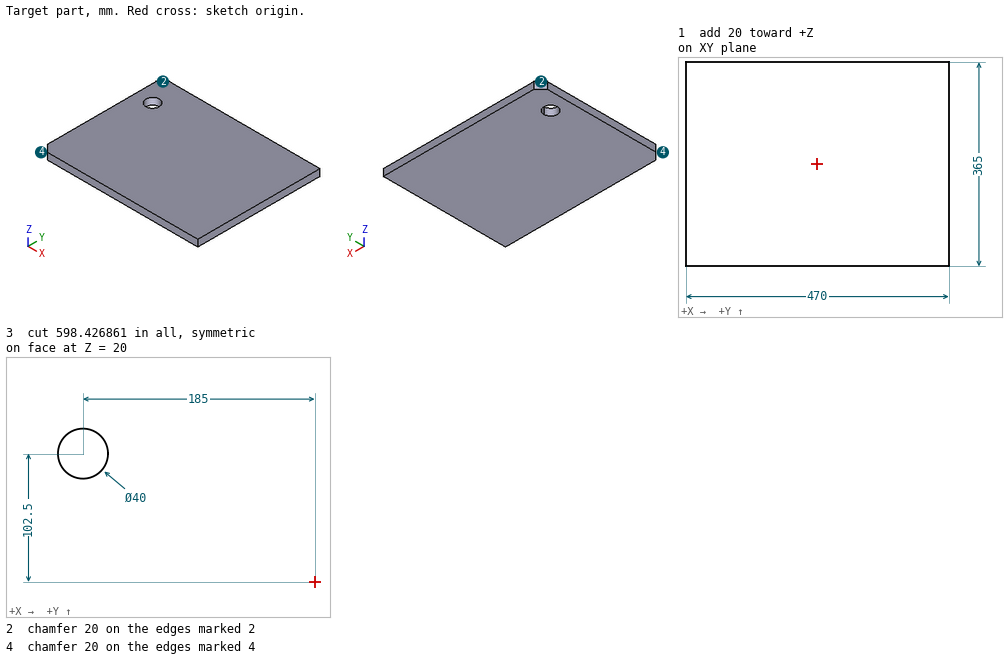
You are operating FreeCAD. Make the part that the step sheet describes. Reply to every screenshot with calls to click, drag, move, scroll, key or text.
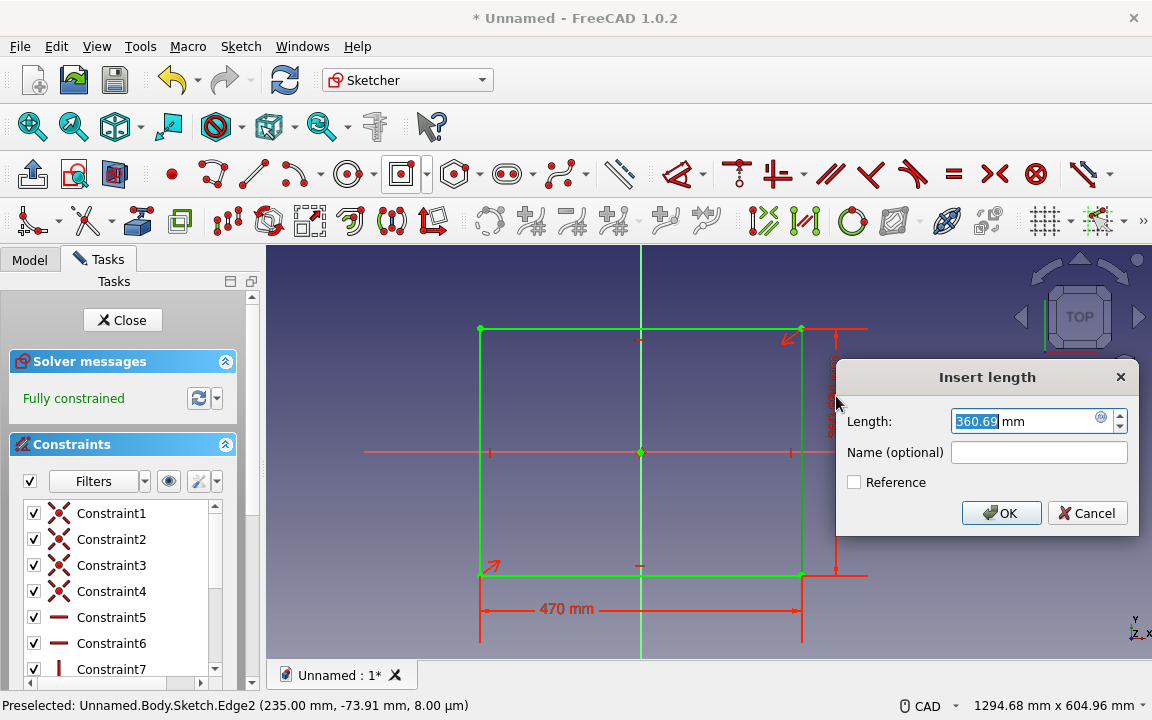
text(365)
key(Return)
key(Escape)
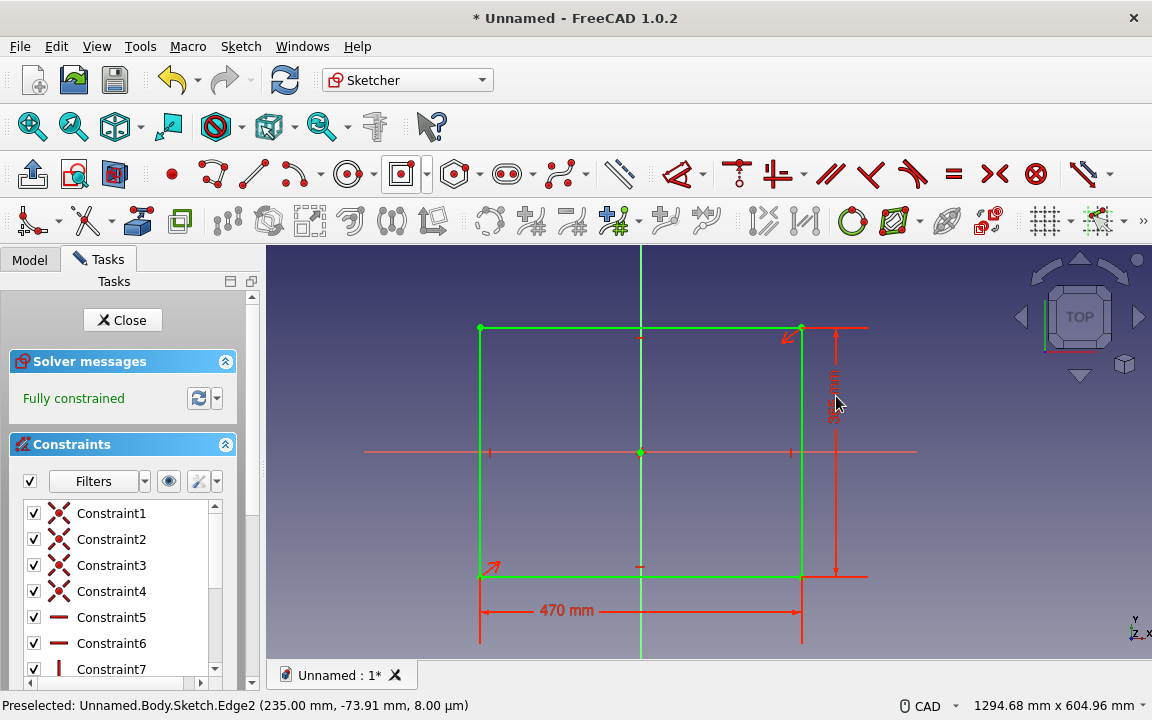
click(123, 320)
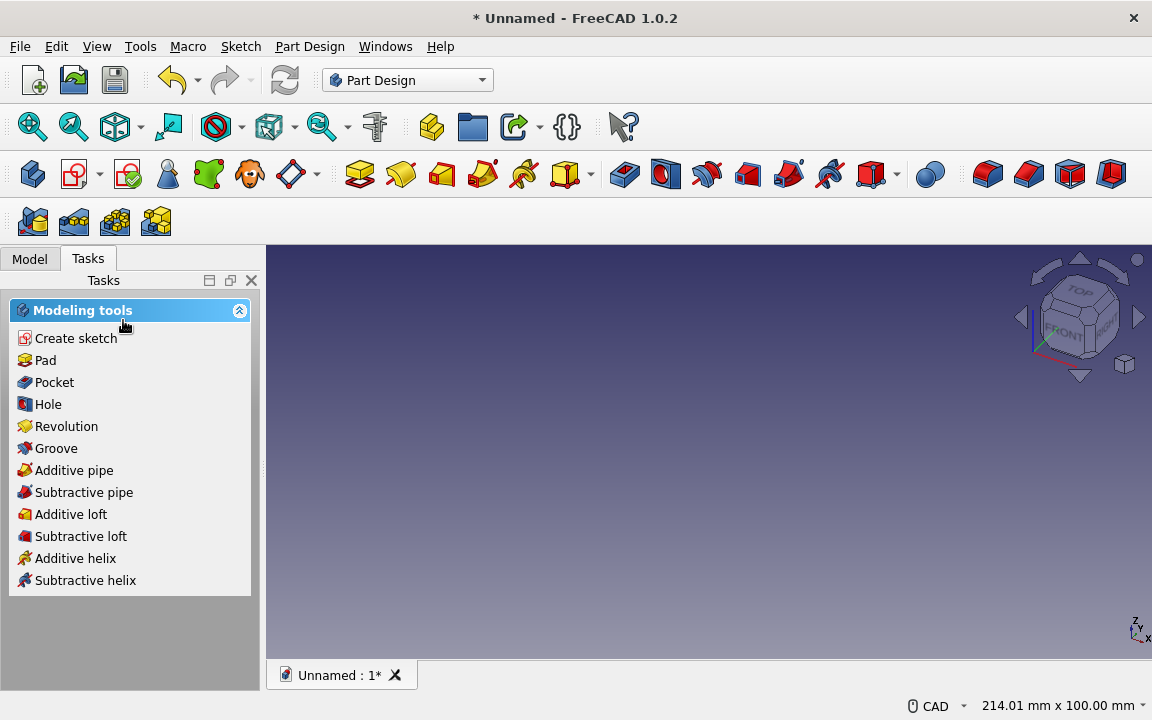
click(360, 174)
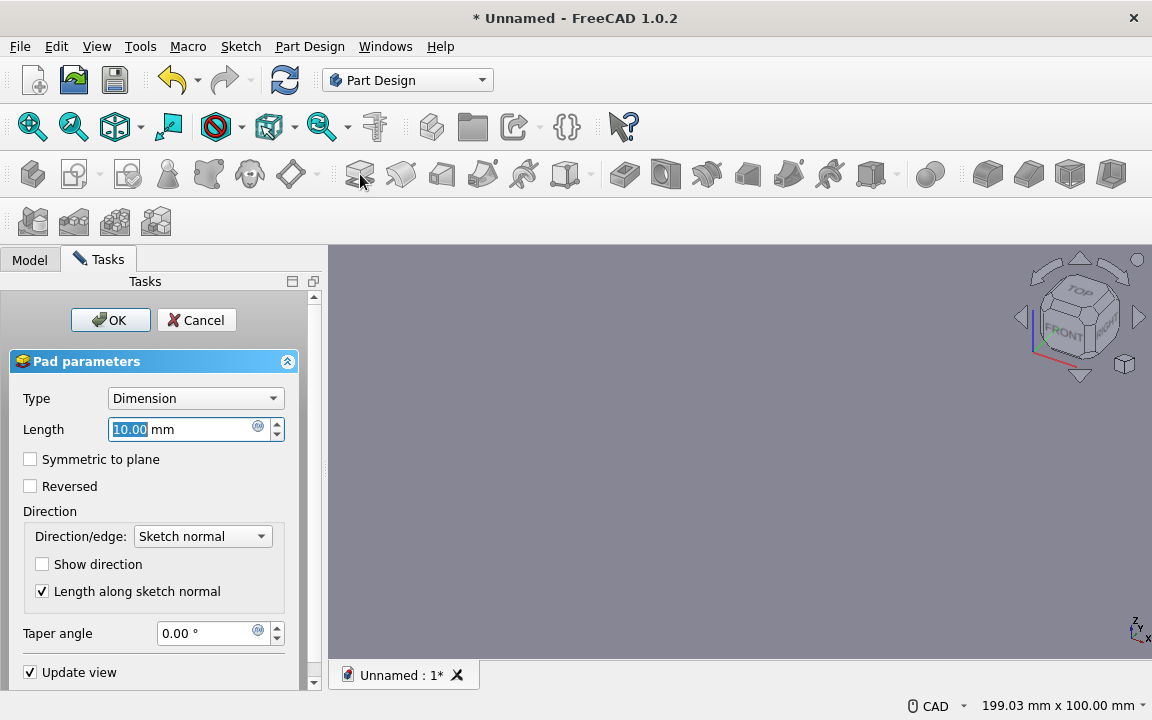
text(20)
key(Tab)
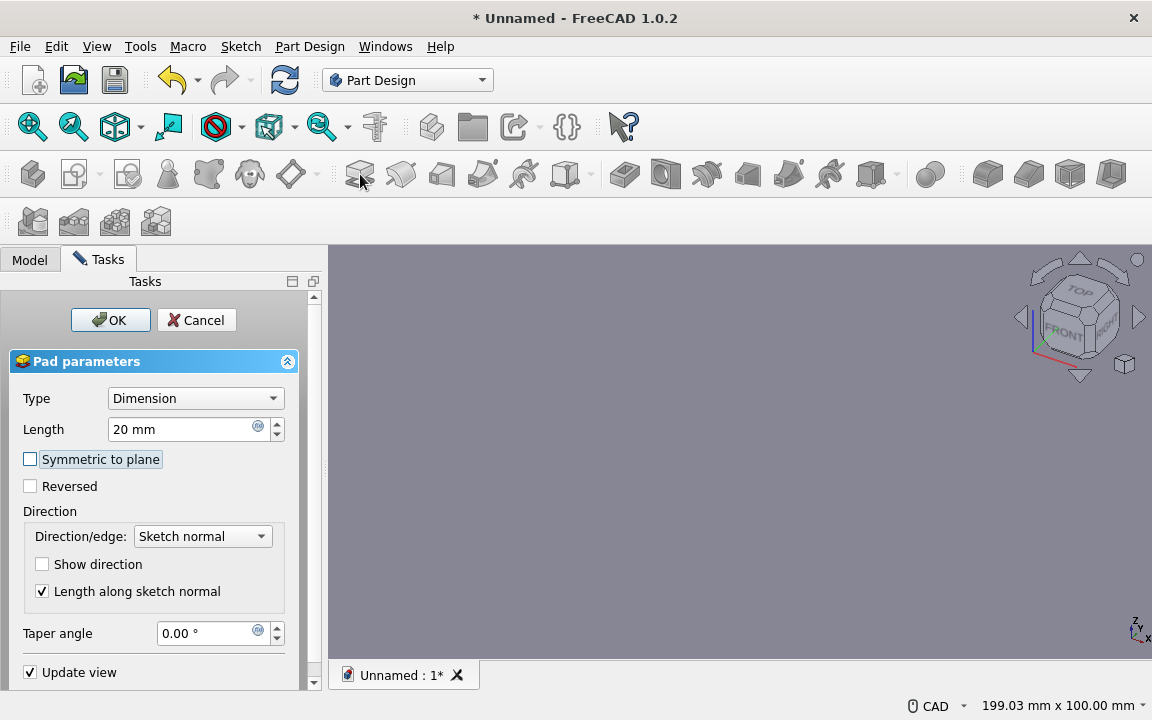
click(111, 320)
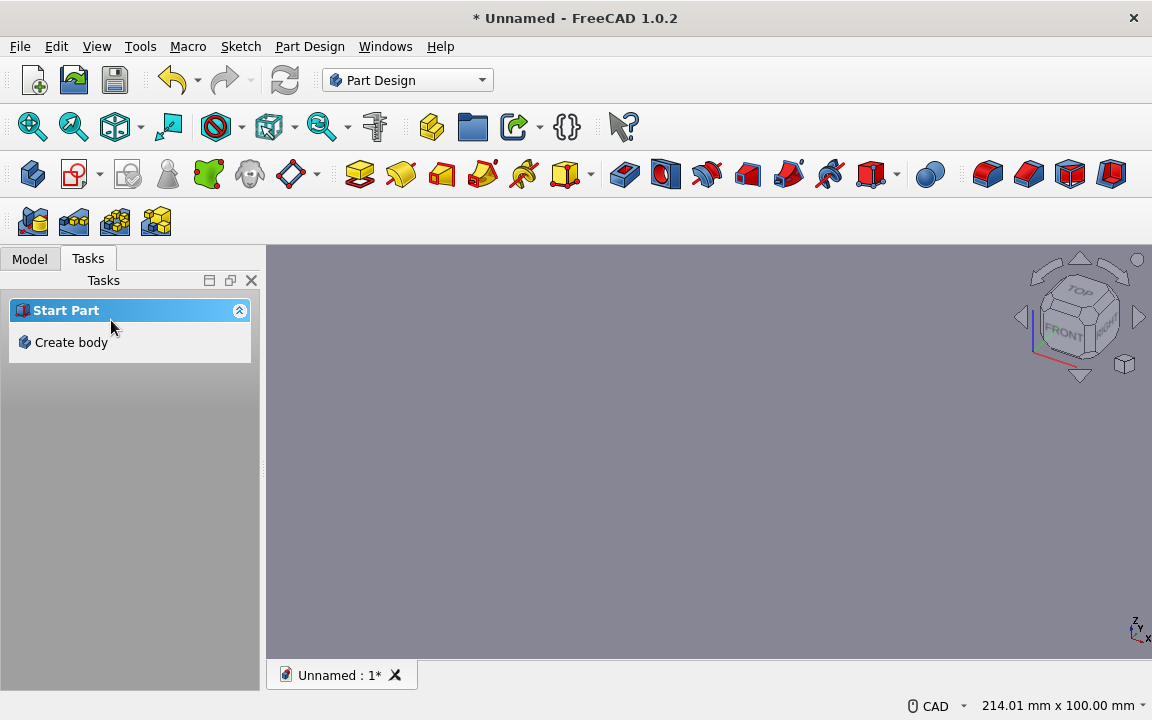
click(33, 128)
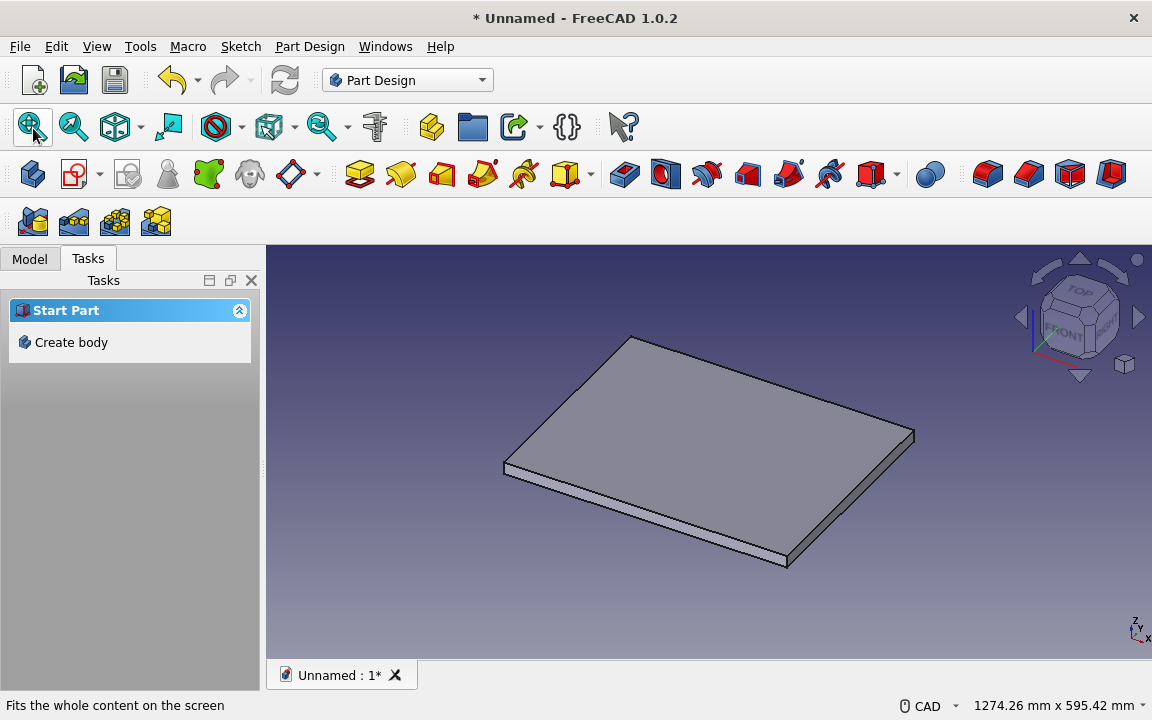
scroll(631, 341, up, 6)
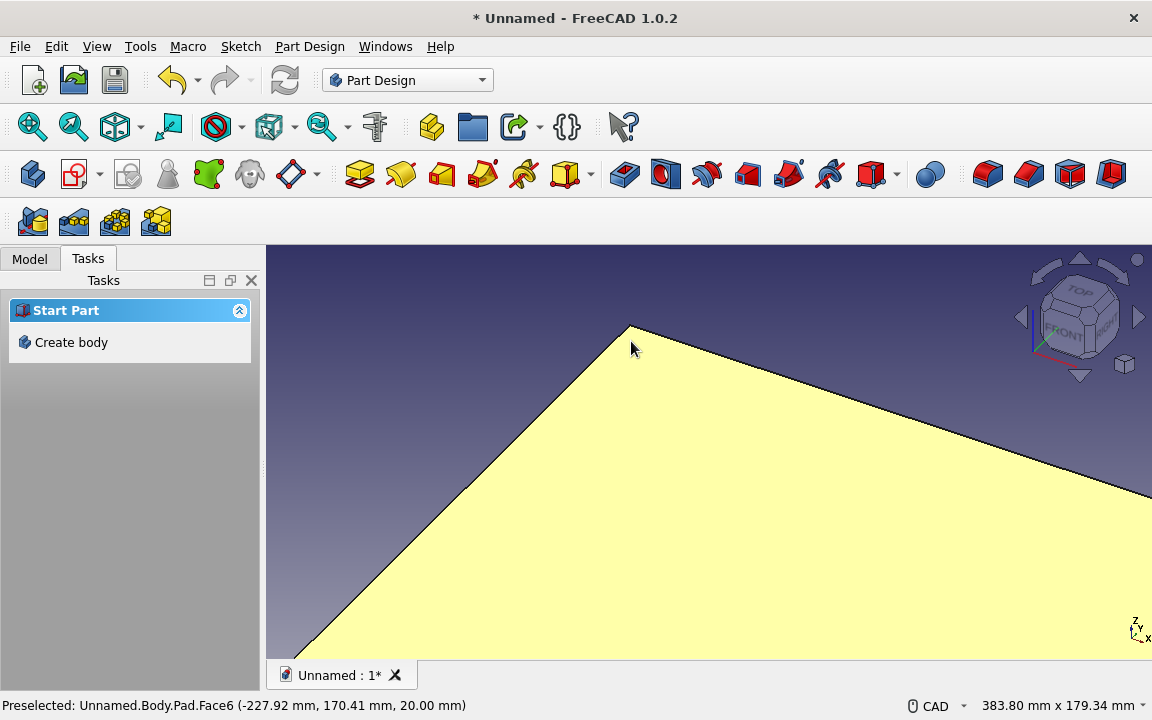
click(33, 128)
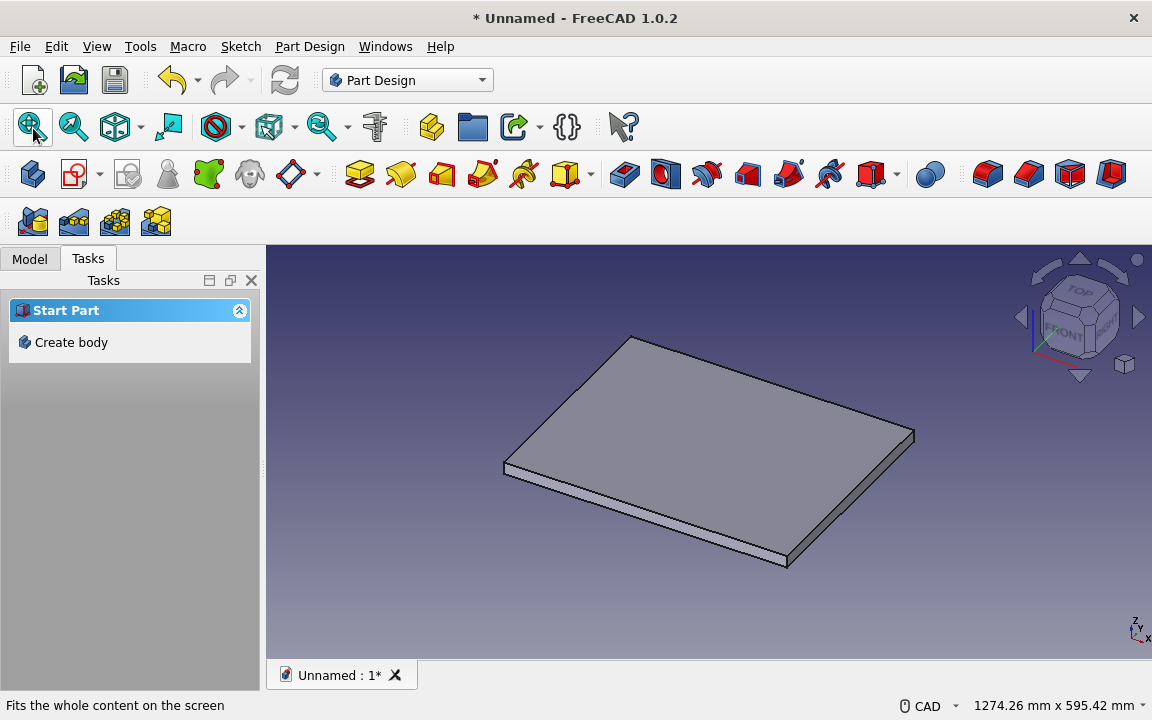
key(0)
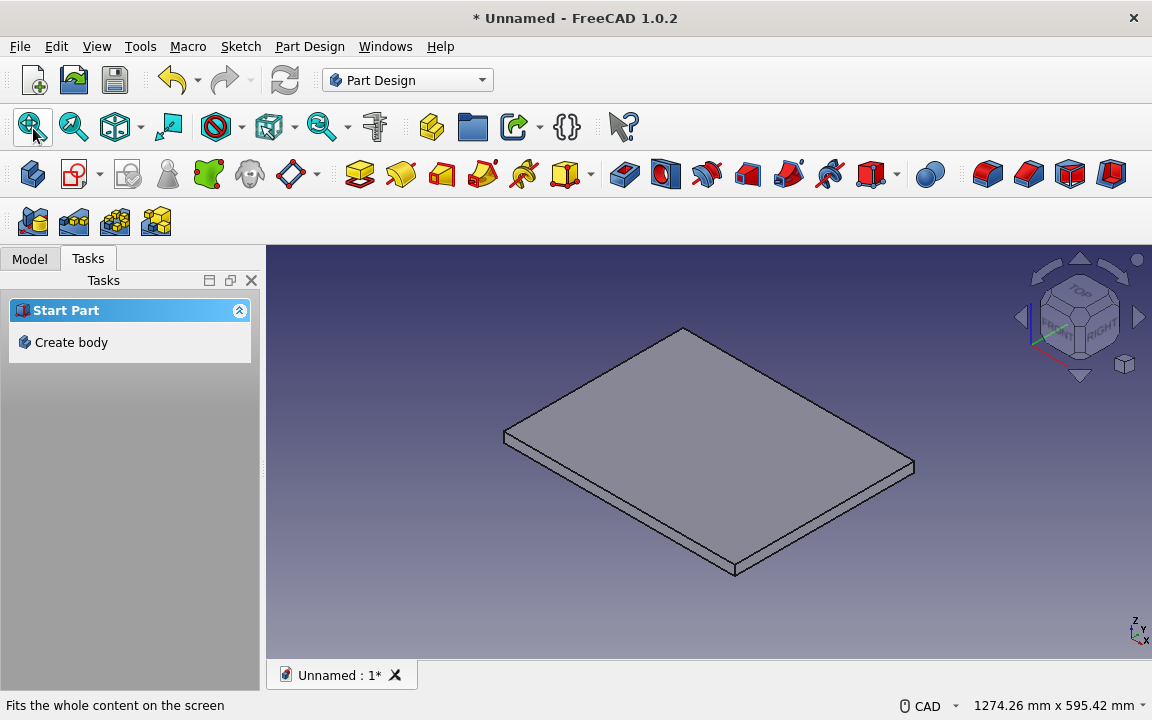
scroll(683, 332, up, 6)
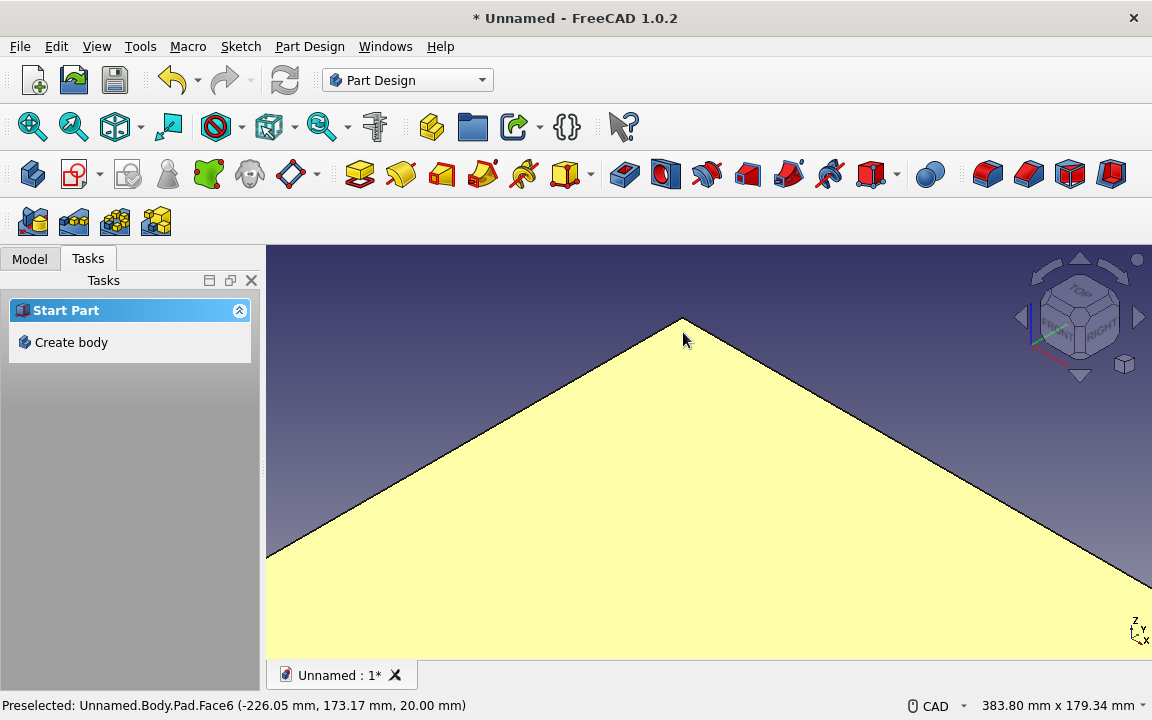
click(33, 128)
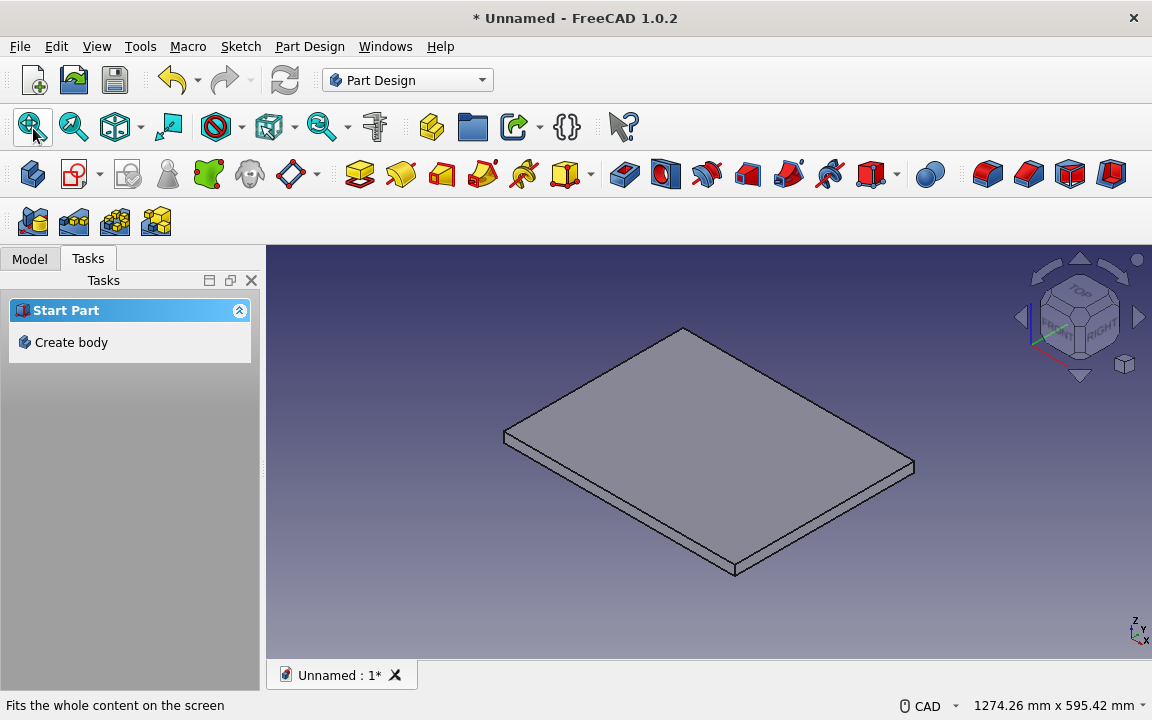
key(2)